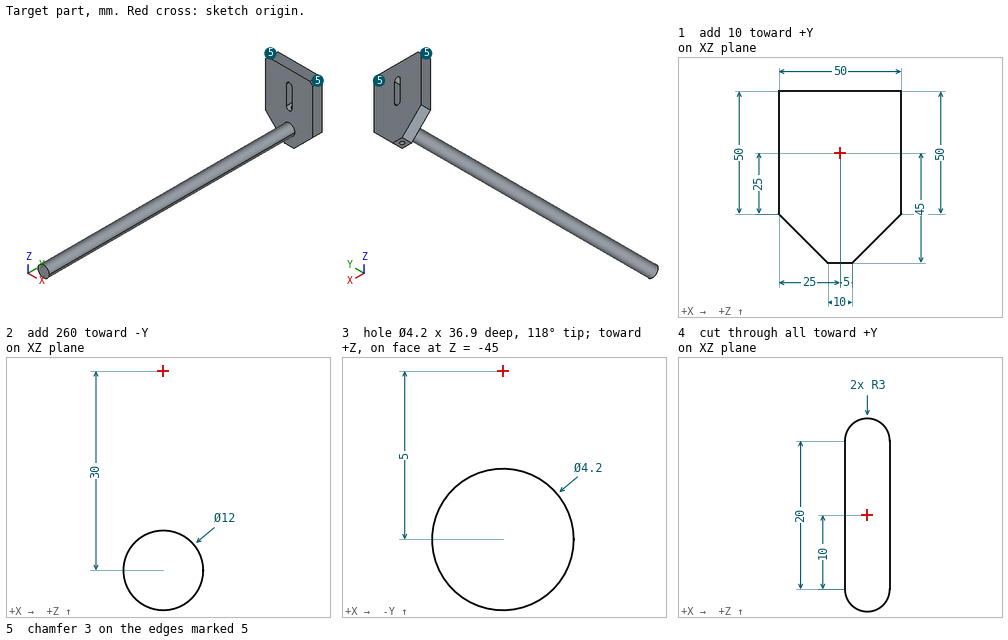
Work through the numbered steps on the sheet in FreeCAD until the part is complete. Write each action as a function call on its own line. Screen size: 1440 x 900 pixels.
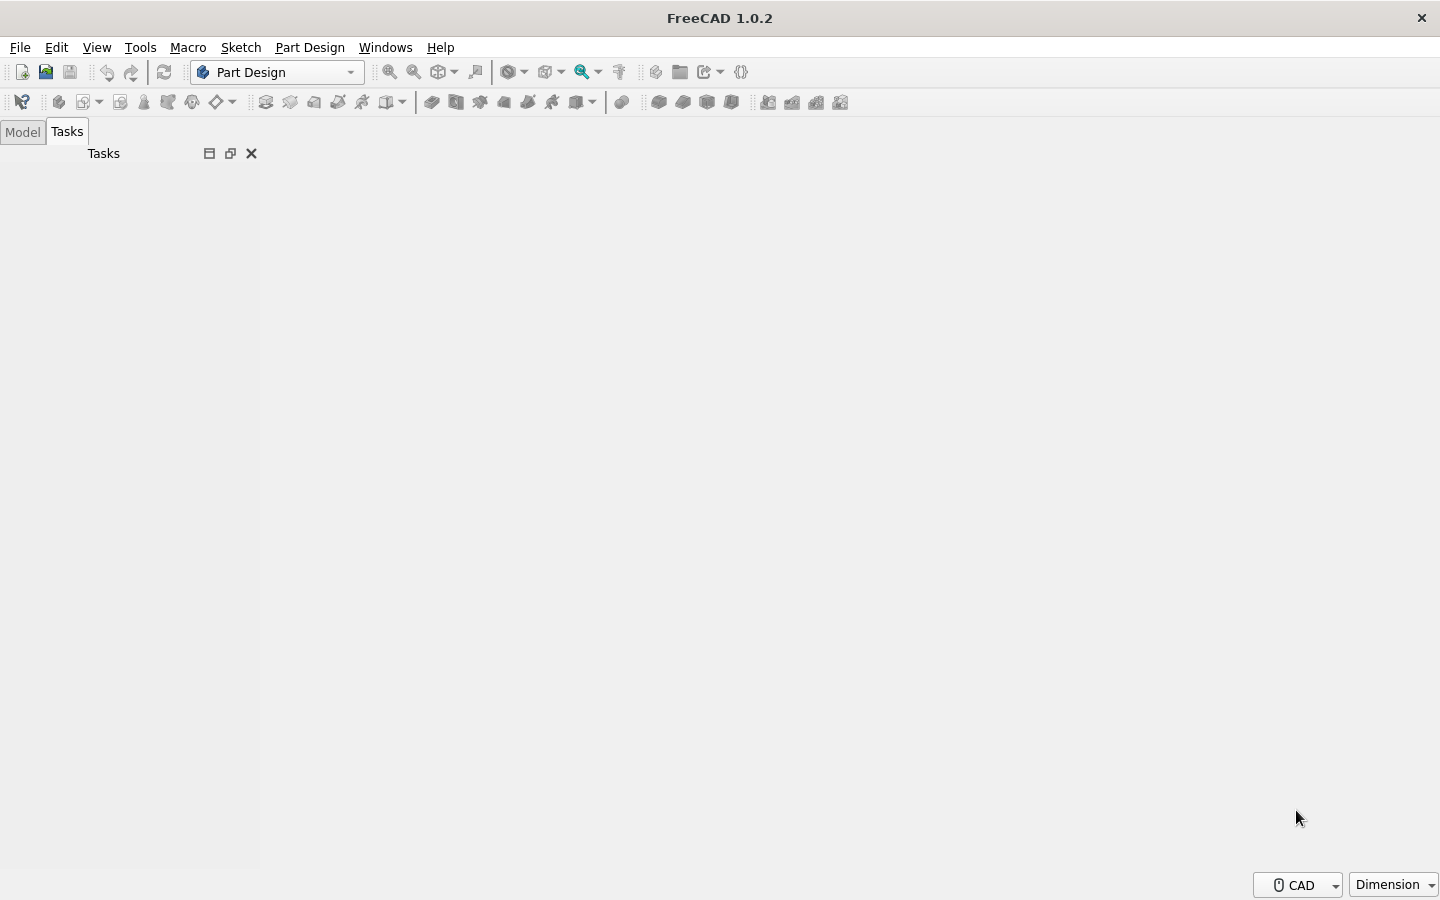
click(22, 72)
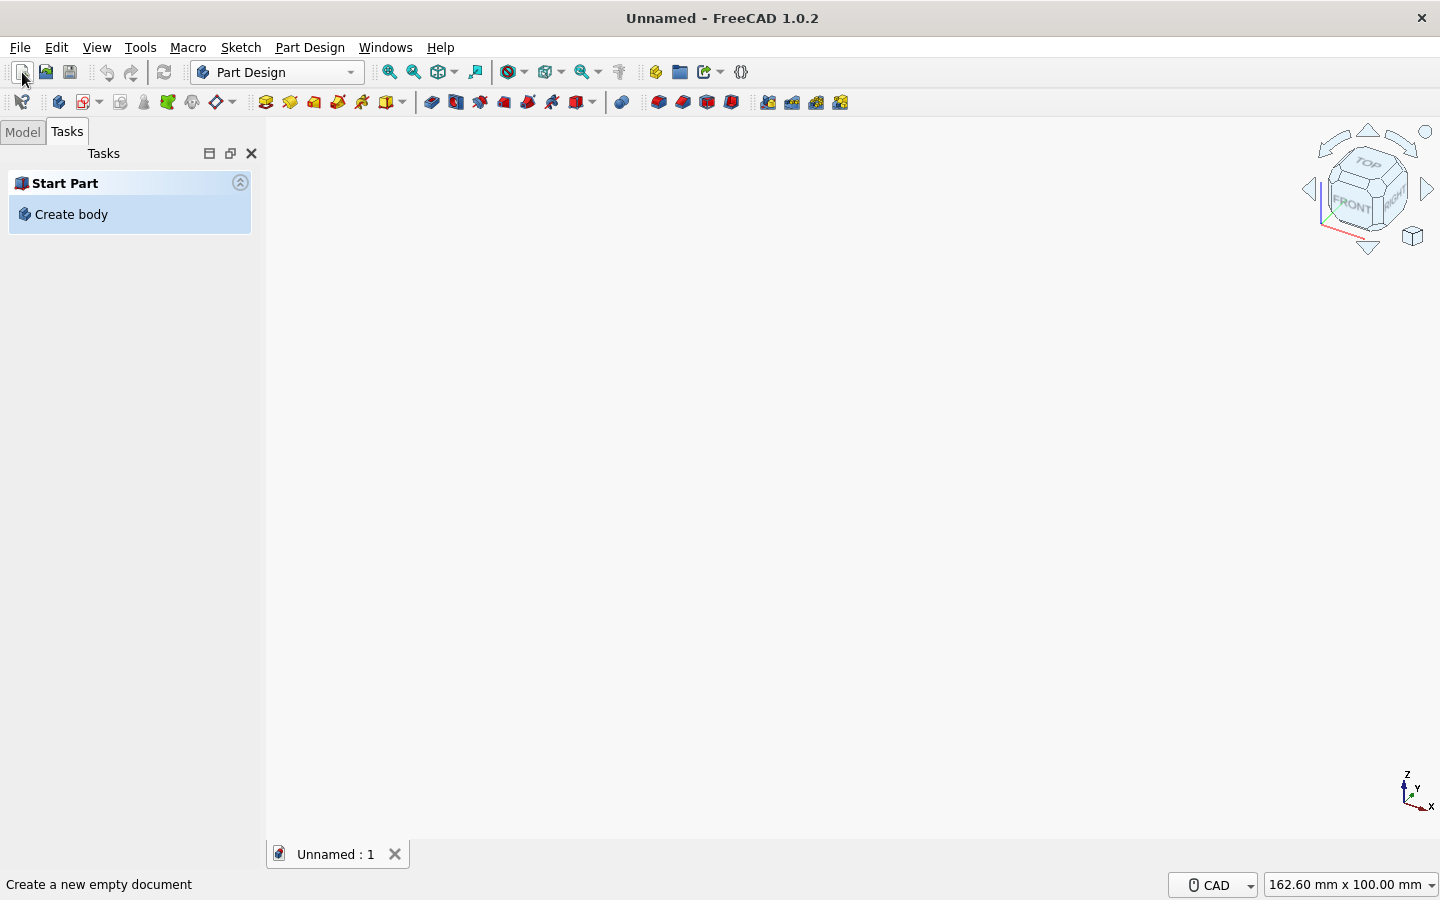
click(84, 102)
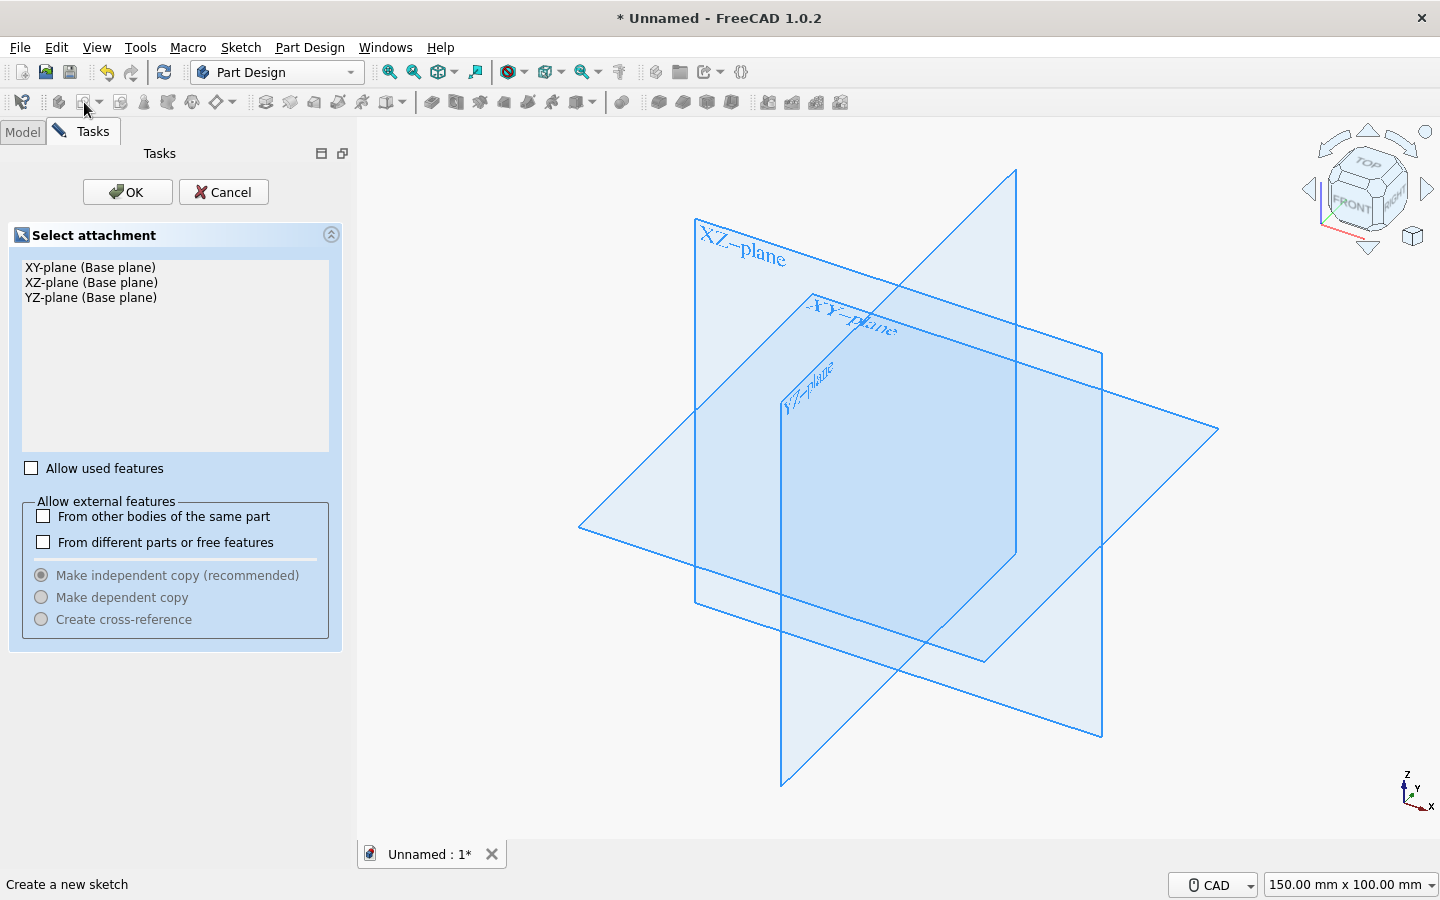
click(82, 282)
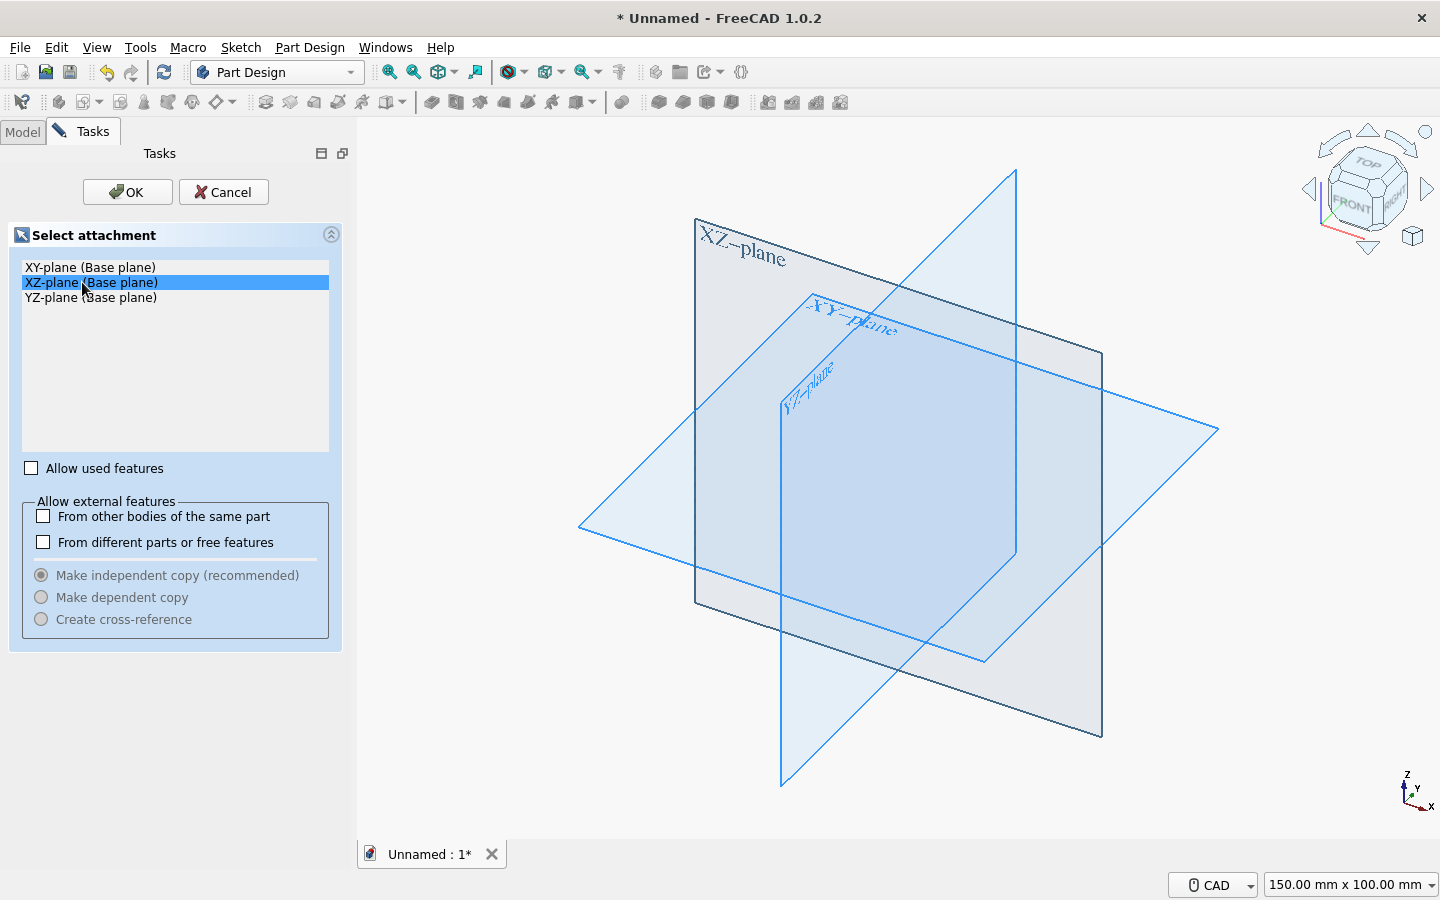
click(128, 192)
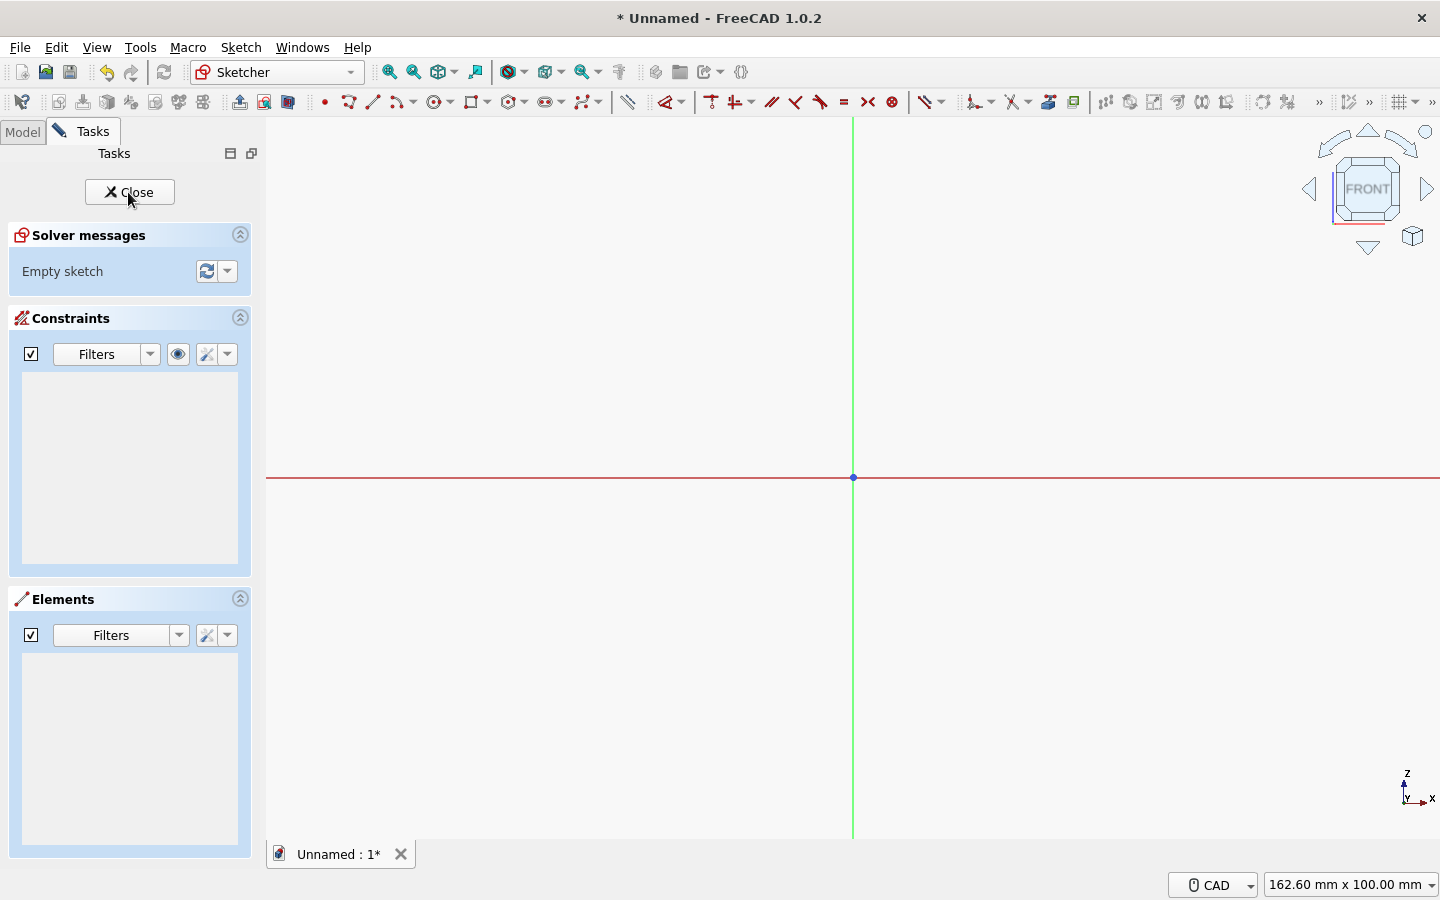
scroll(475, 152, down, 1)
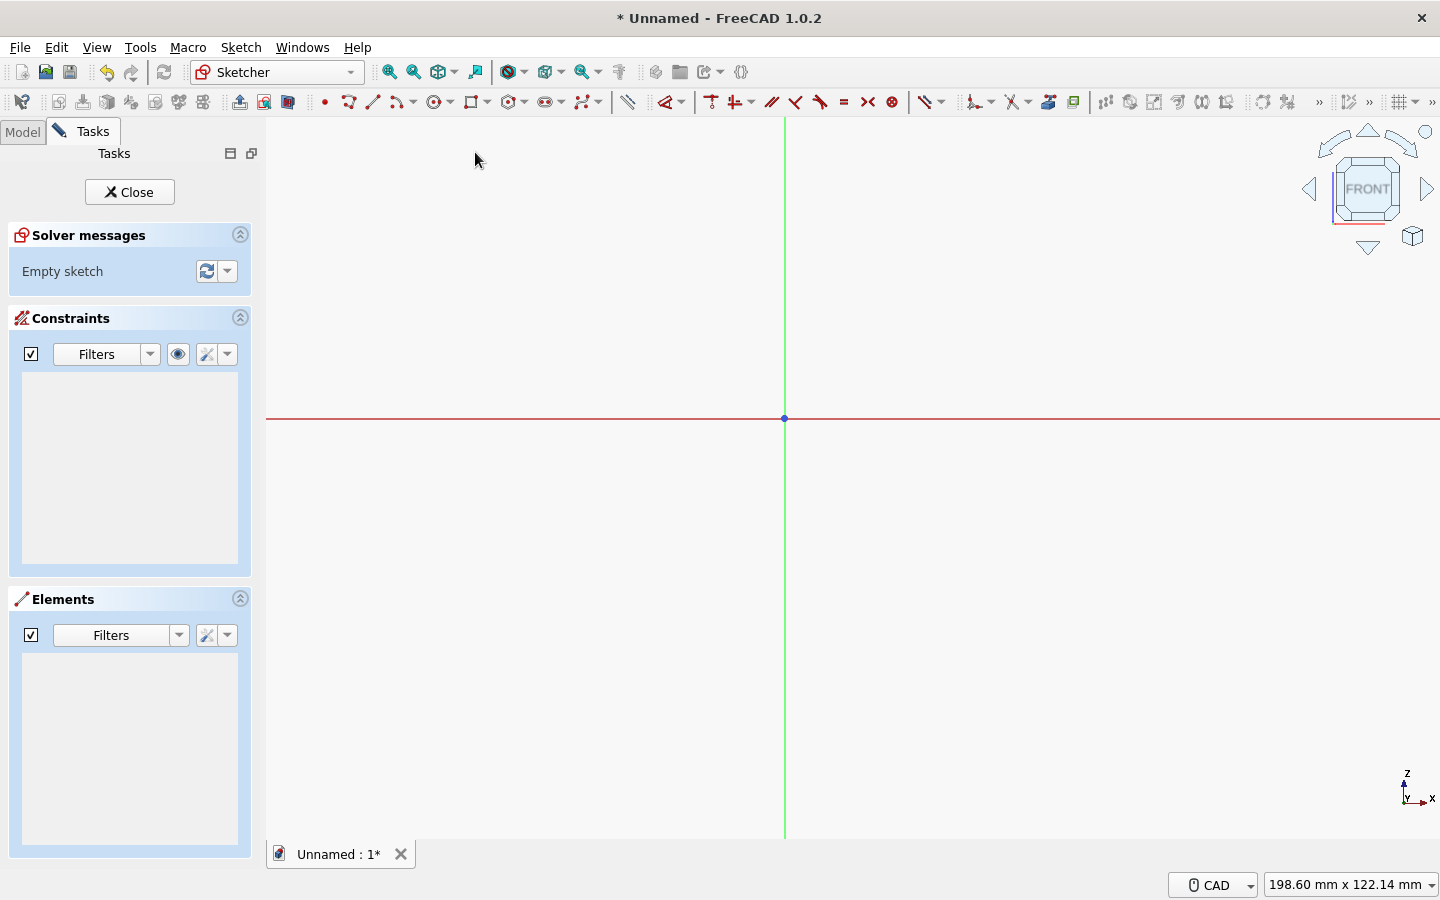
click(350, 102)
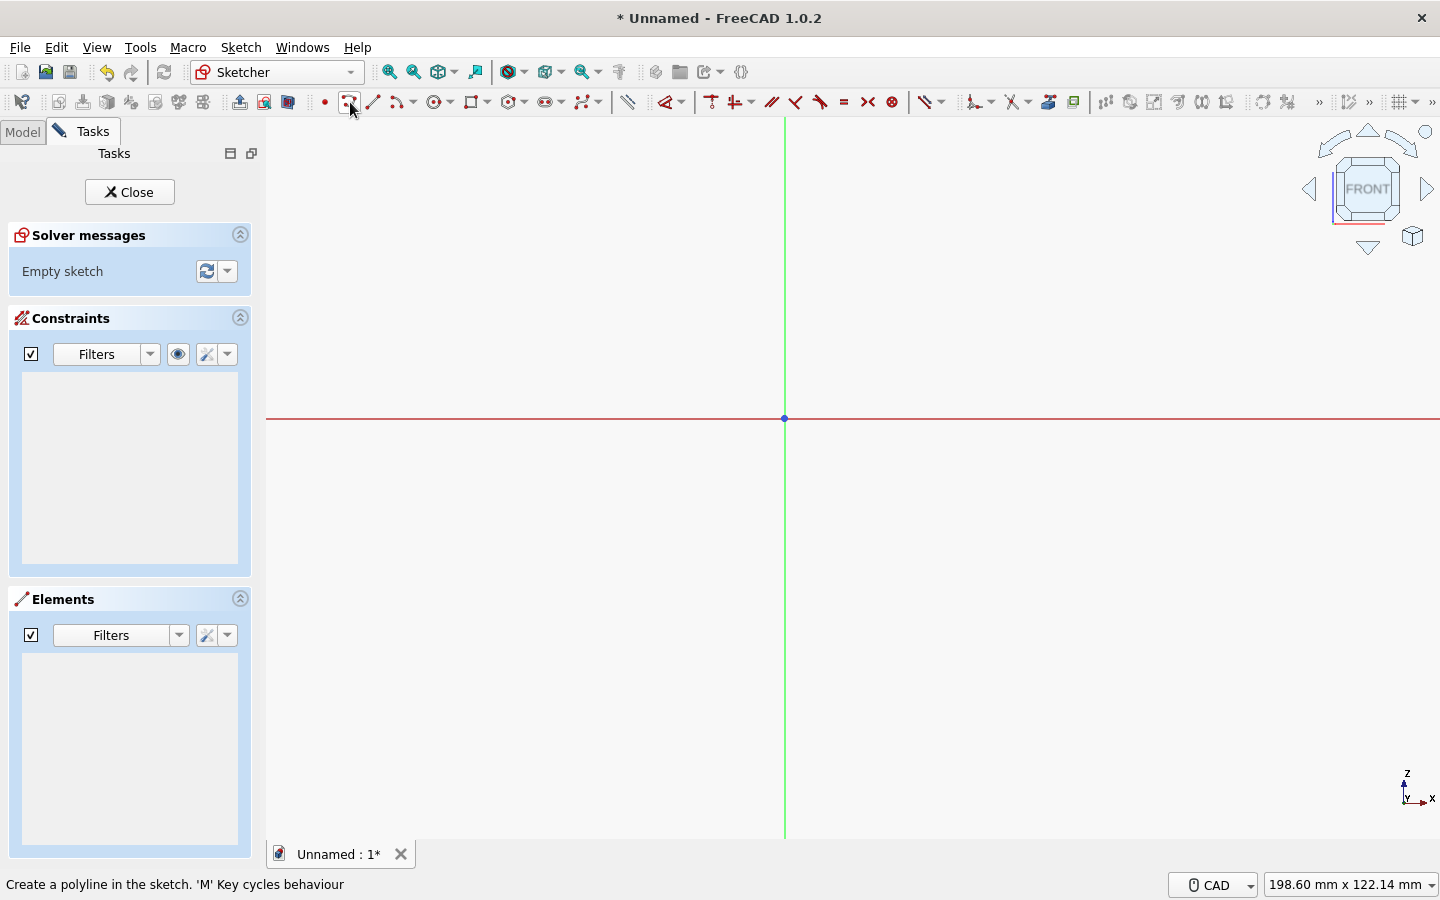
click(637, 567)
click(637, 271)
click(932, 271)
click(932, 567)
click(814, 685)
click(755, 685)
click(637, 568)
key(Escape)
key(Escape)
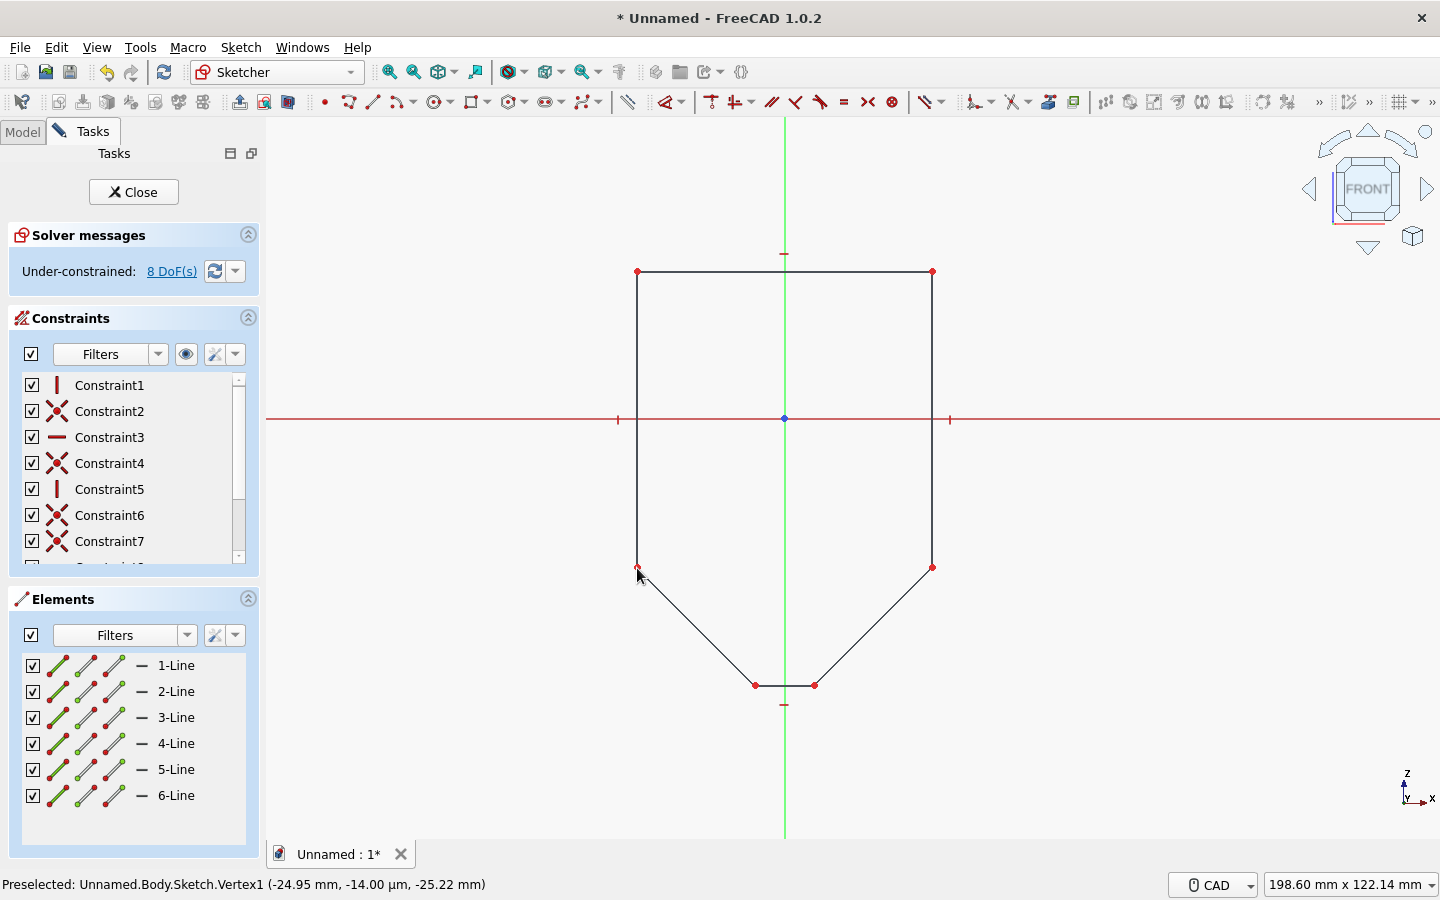
click(666, 102)